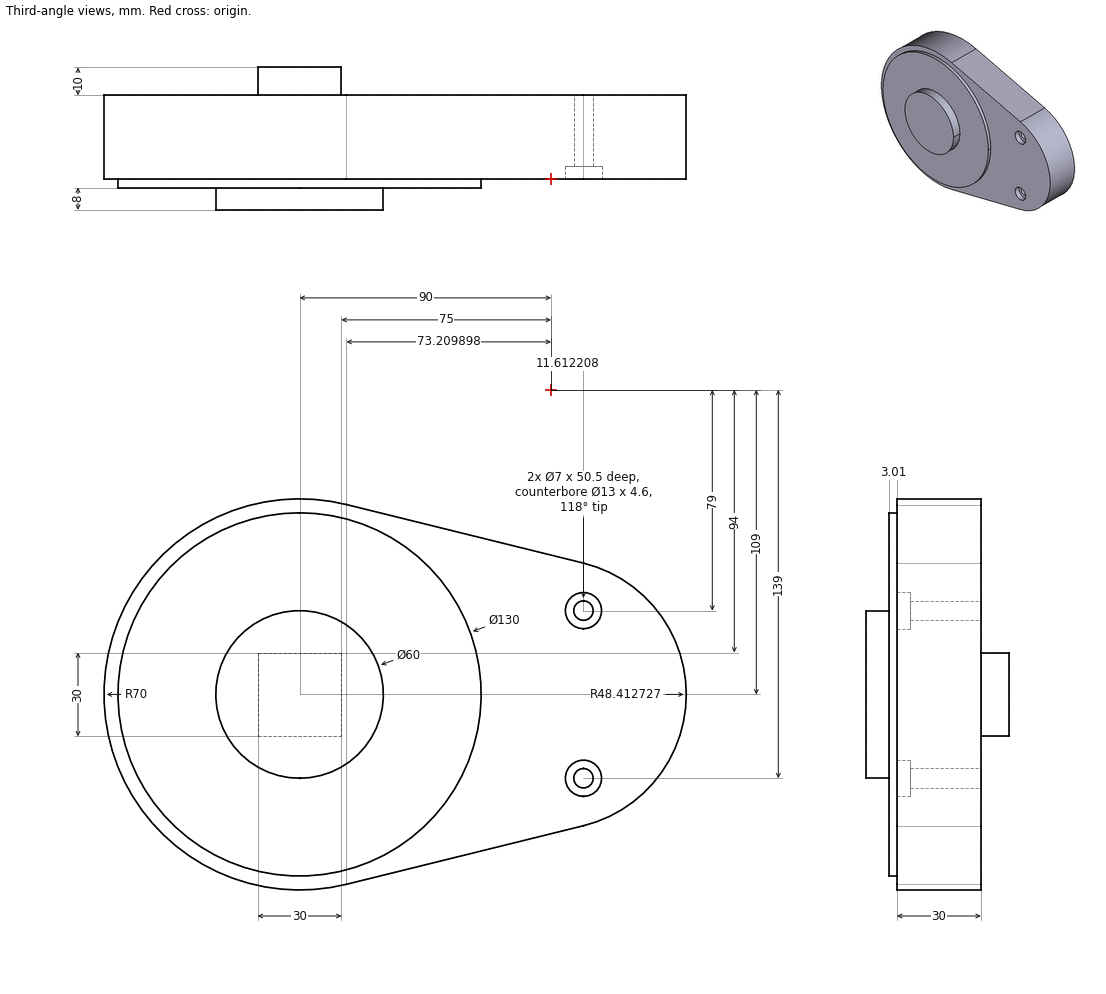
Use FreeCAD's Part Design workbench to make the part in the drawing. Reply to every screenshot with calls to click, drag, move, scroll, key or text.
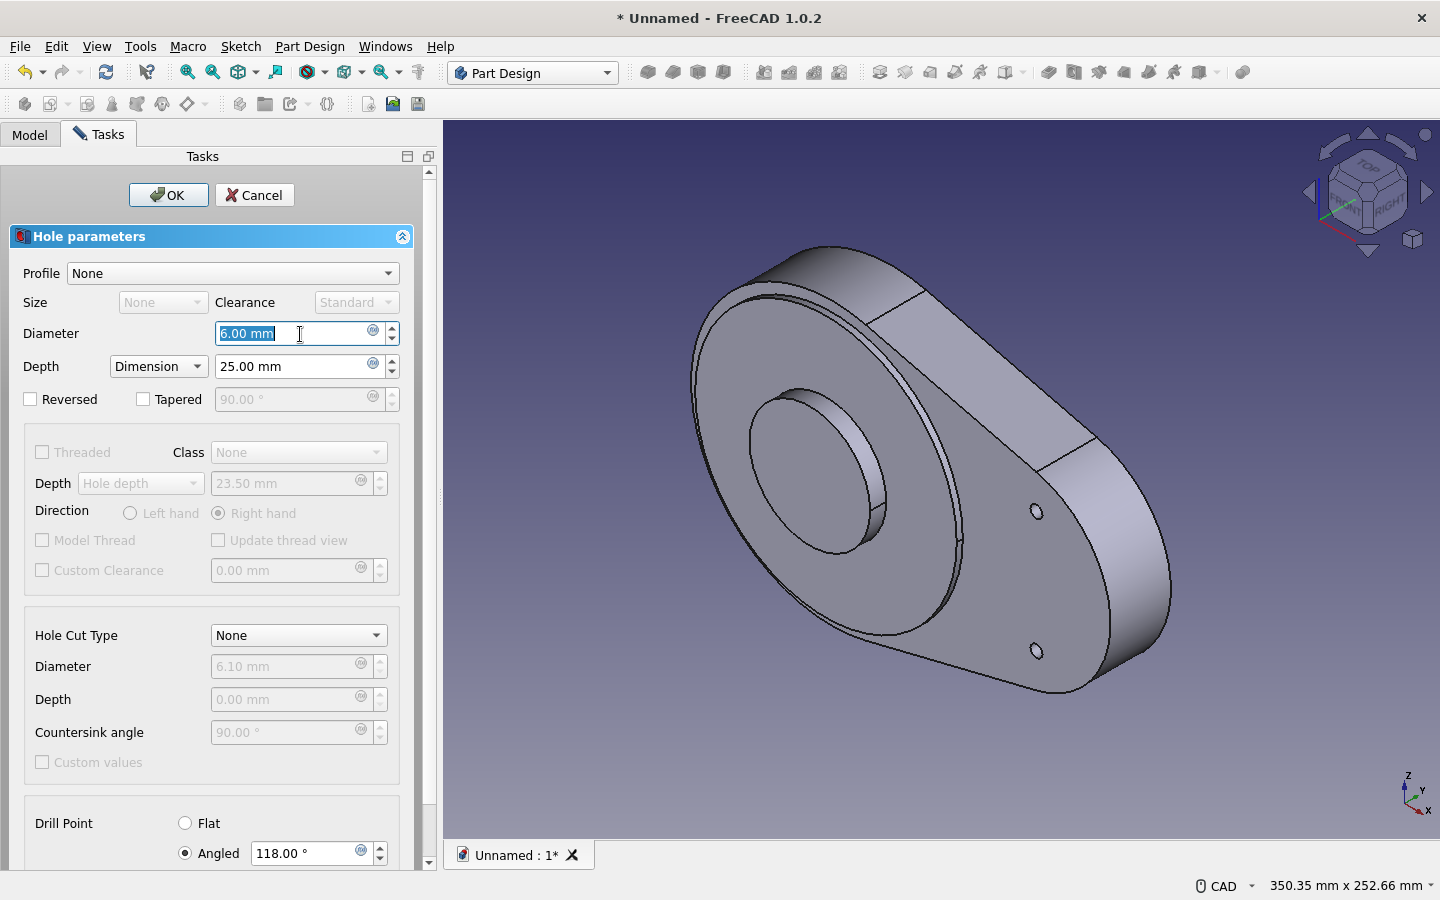
text(7)
key(Tab)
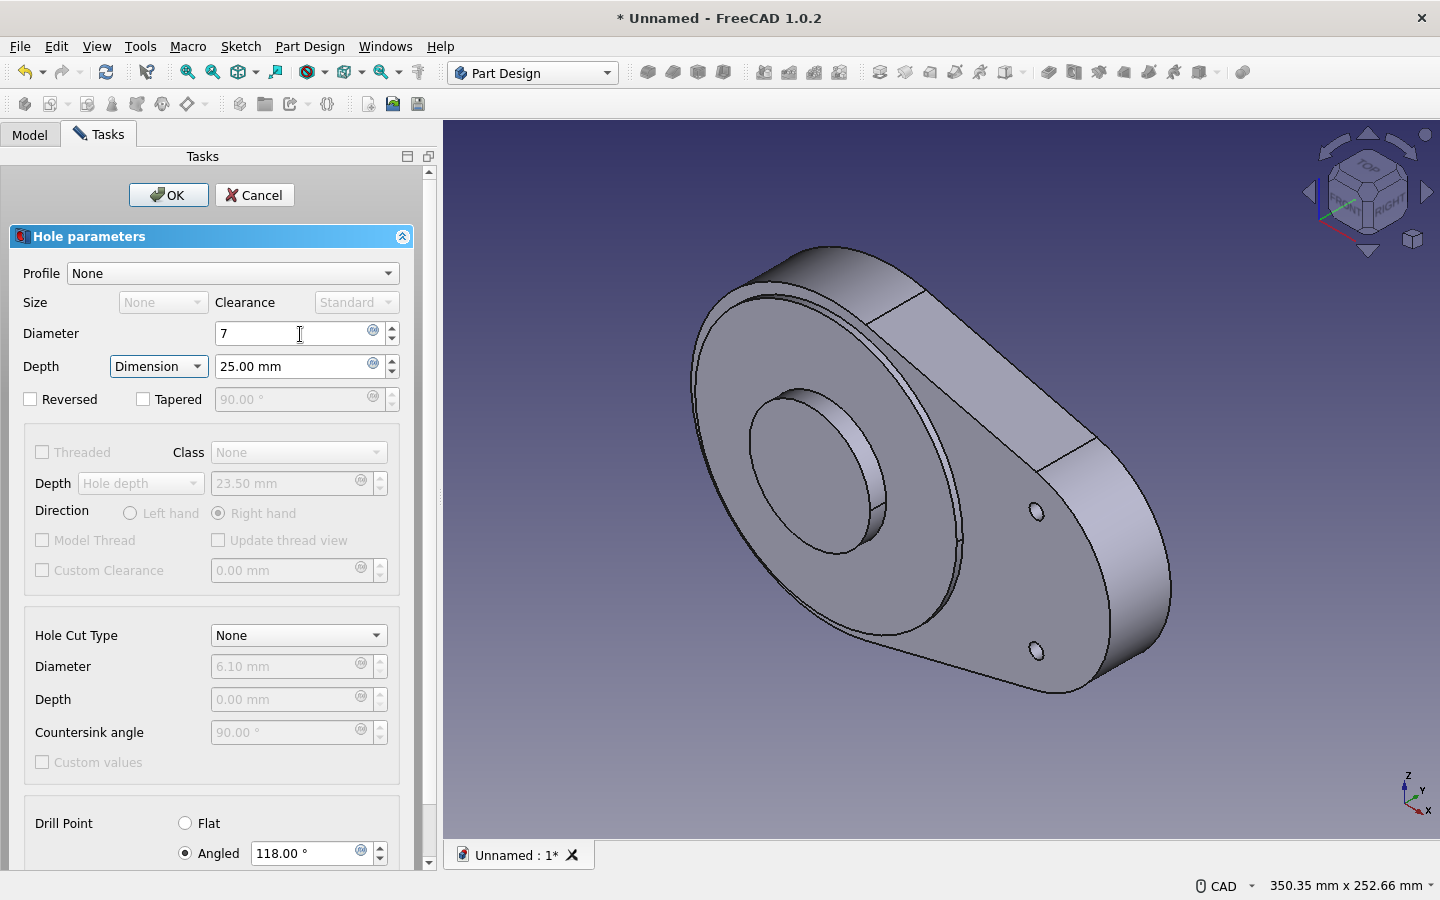
triple_click(300, 366)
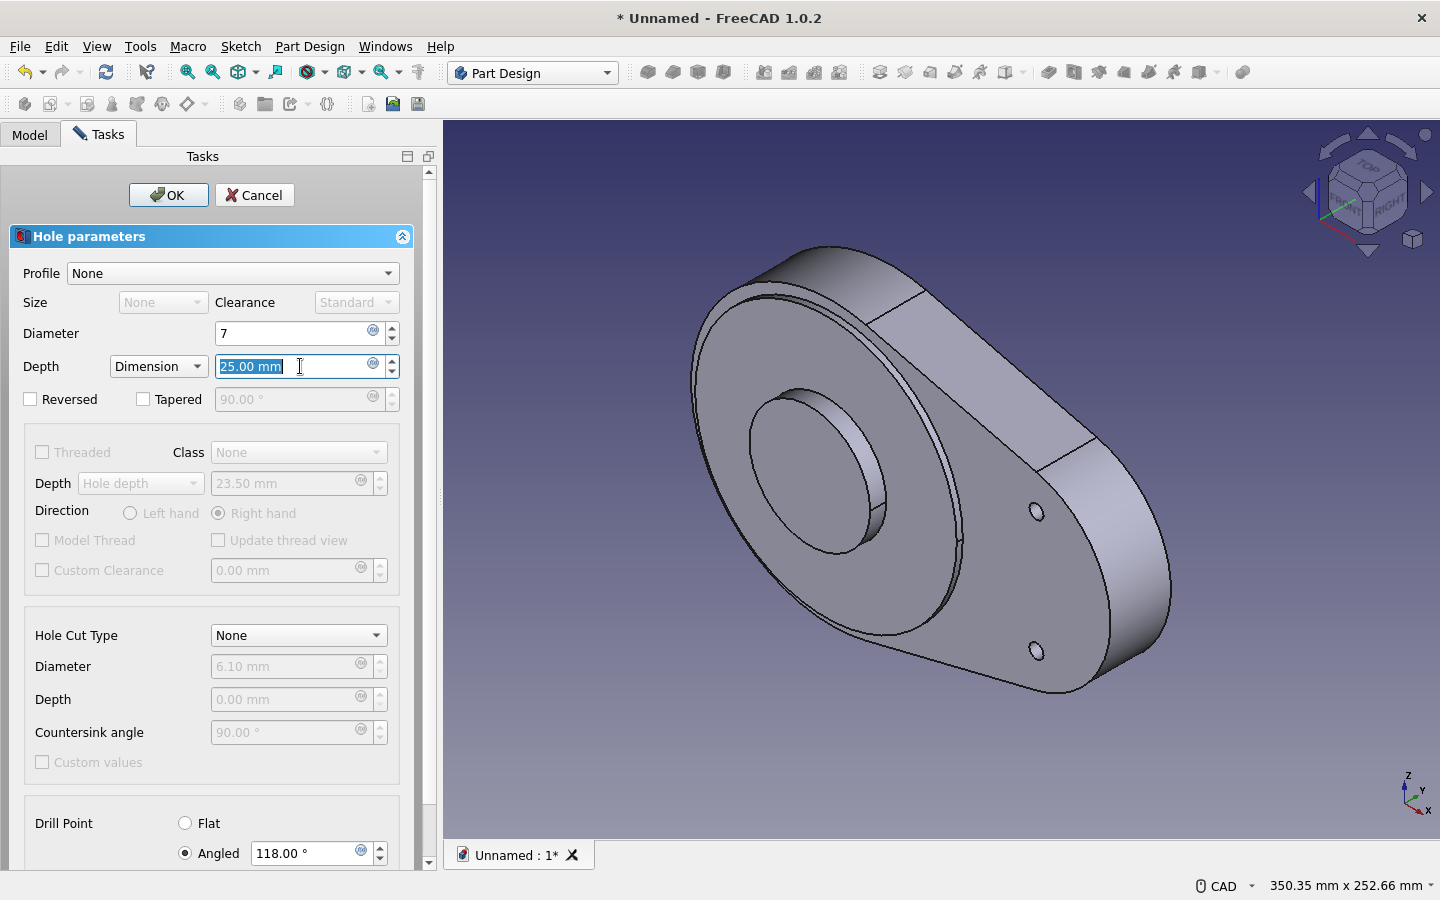
text(50.5)
key(Tab)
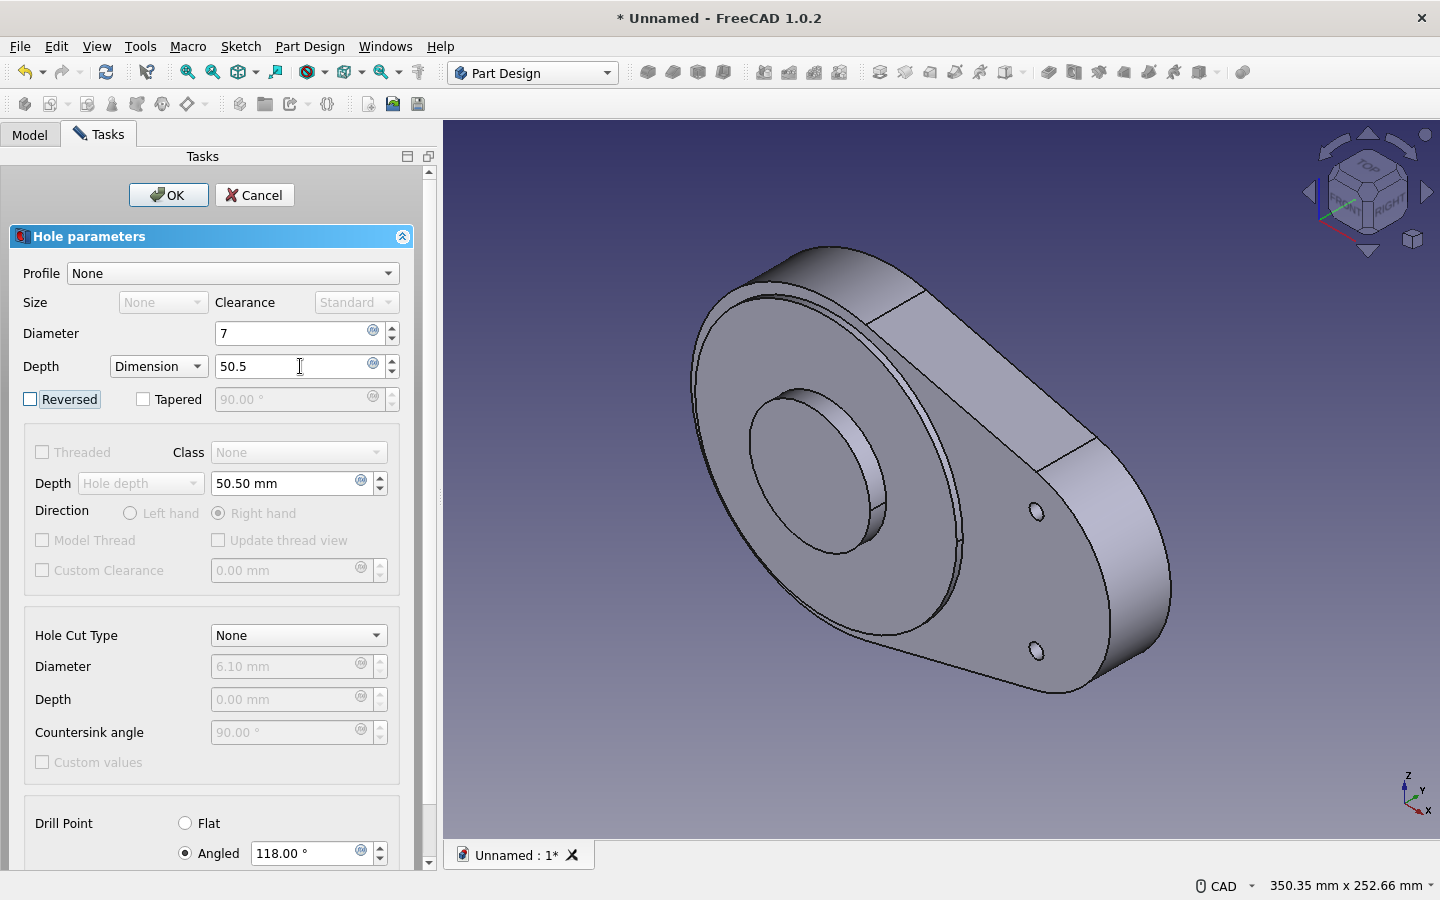
click(300, 636)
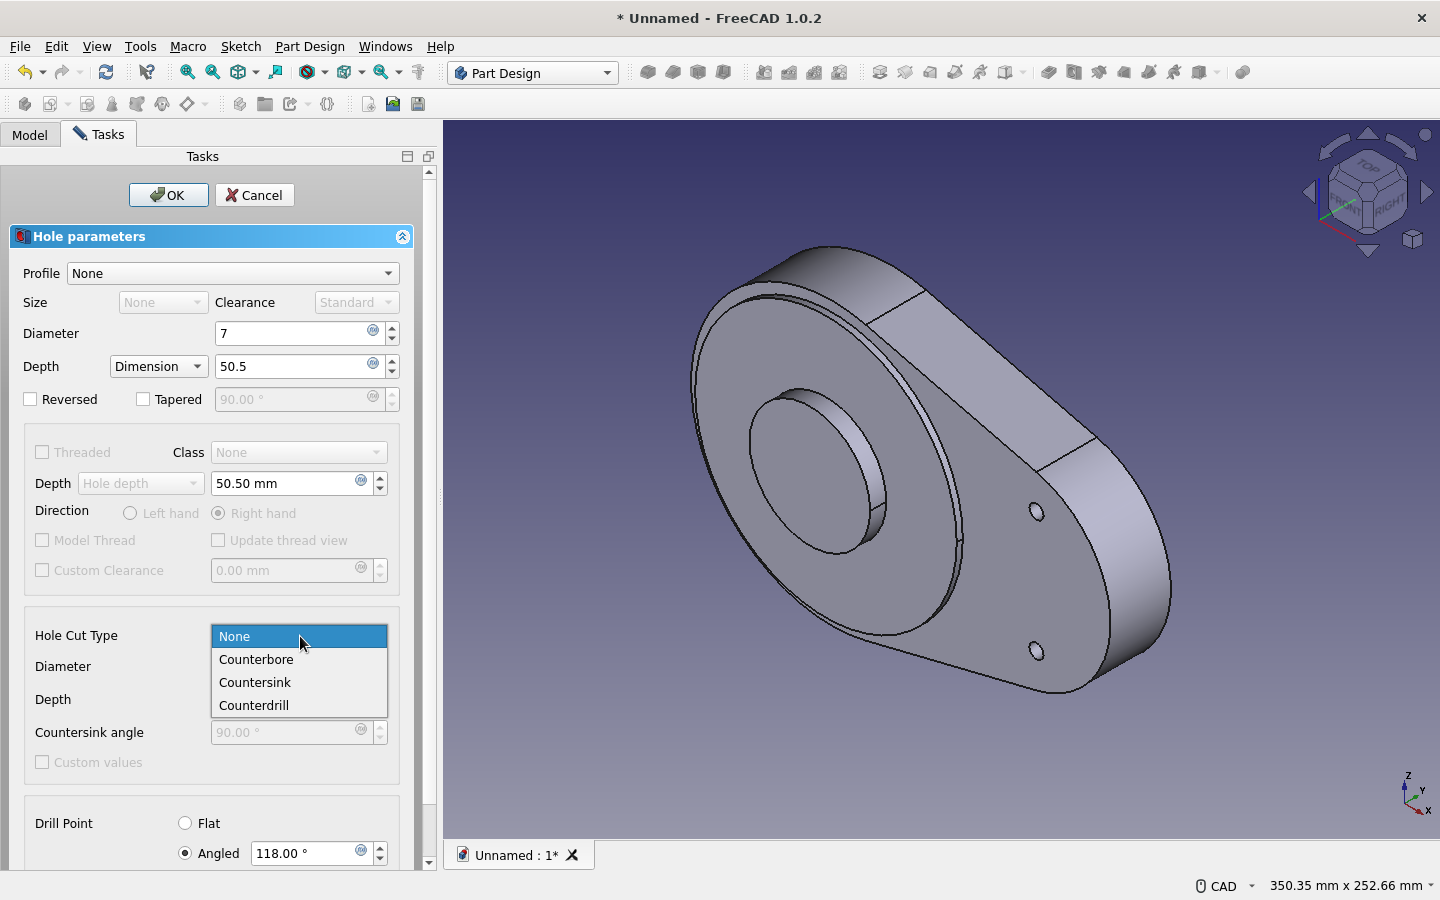
click(298, 660)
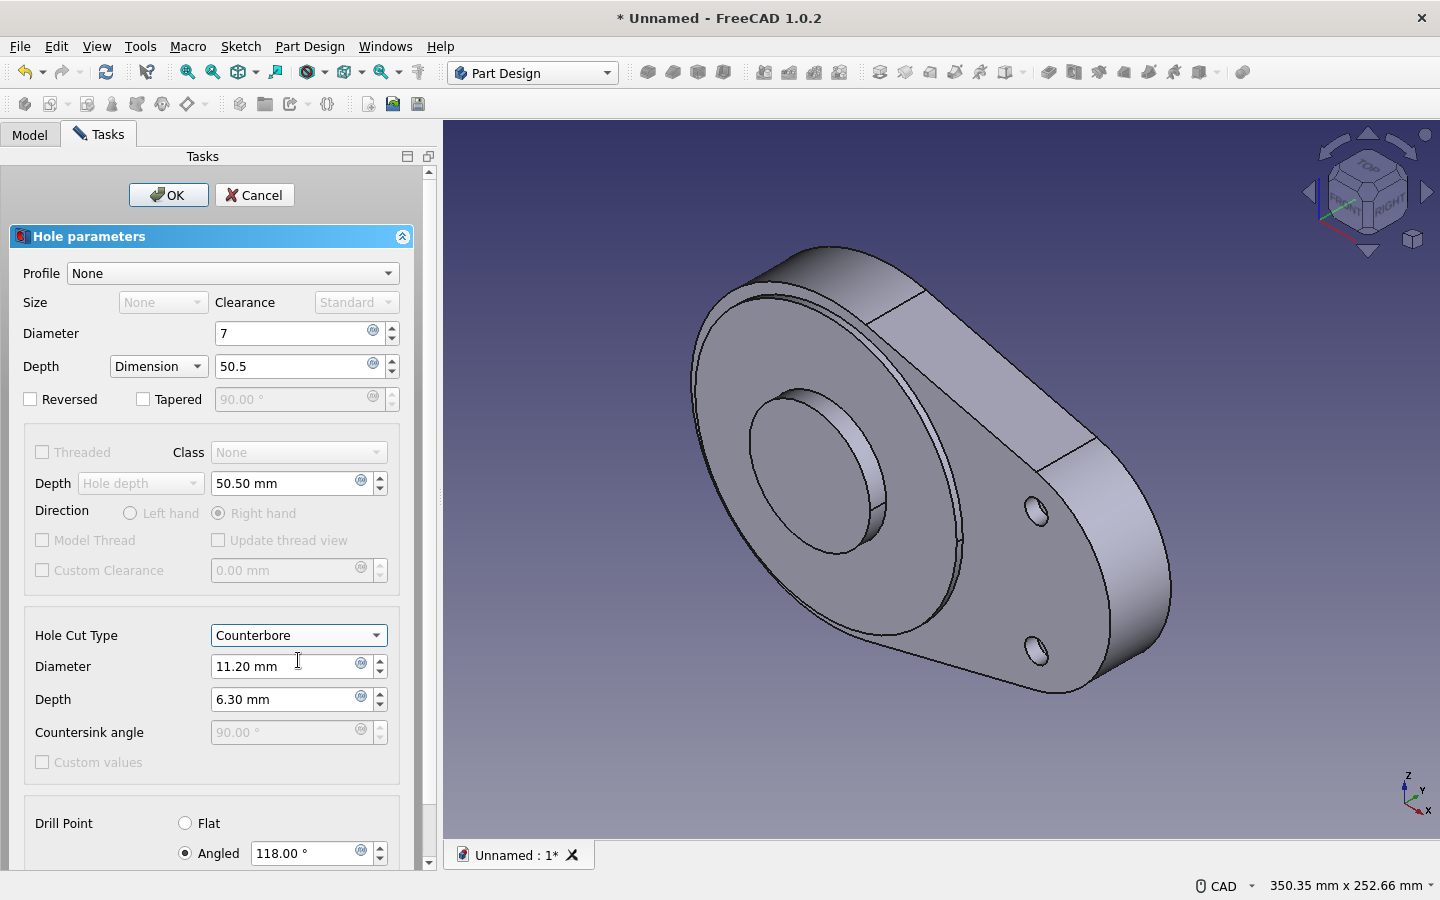
triple_click(292, 666)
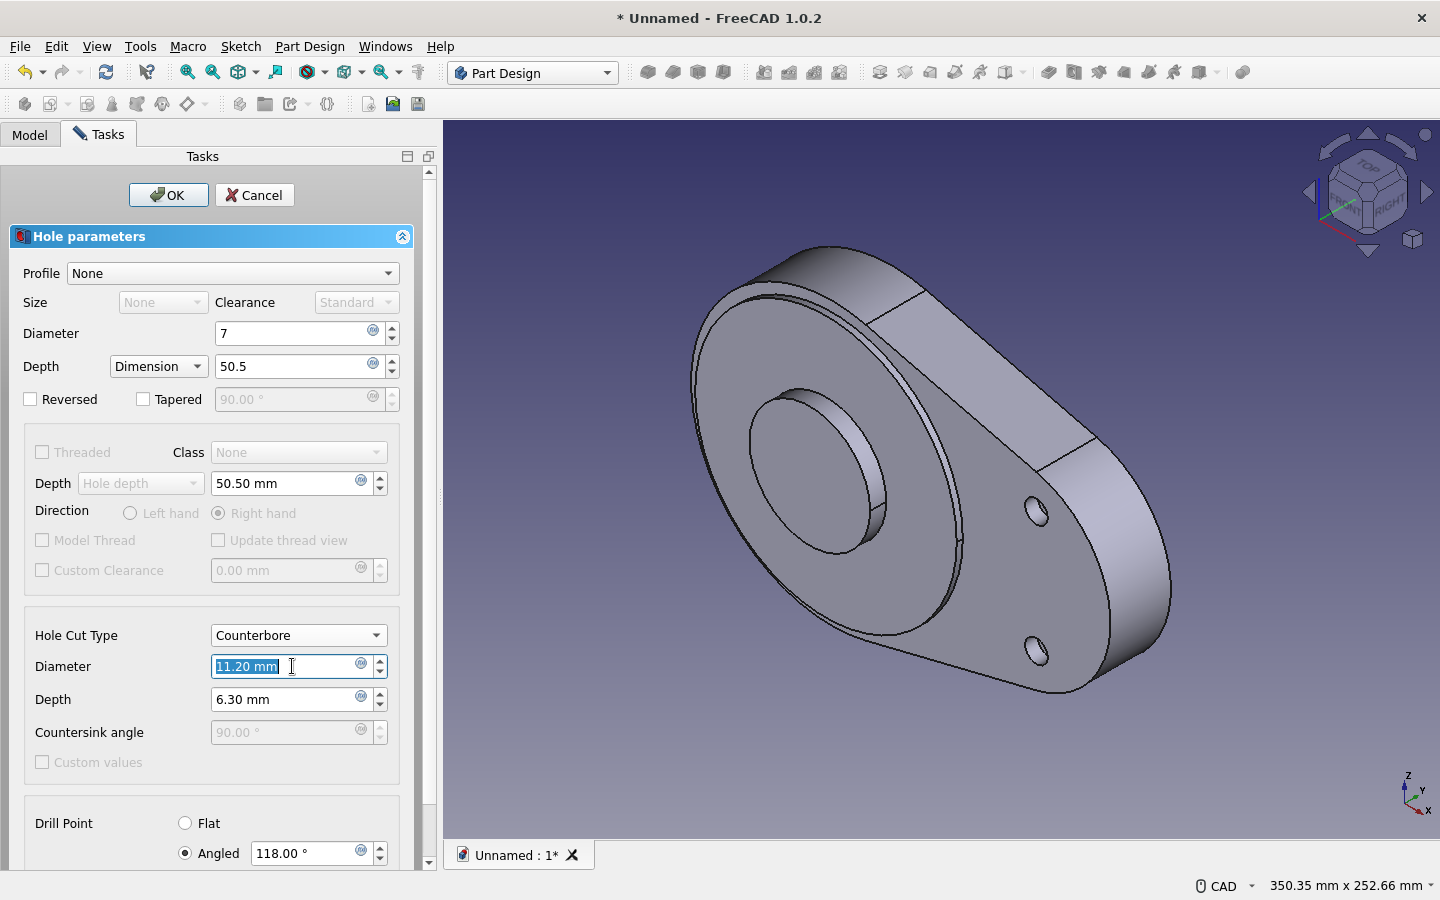
text(13)
key(Tab)